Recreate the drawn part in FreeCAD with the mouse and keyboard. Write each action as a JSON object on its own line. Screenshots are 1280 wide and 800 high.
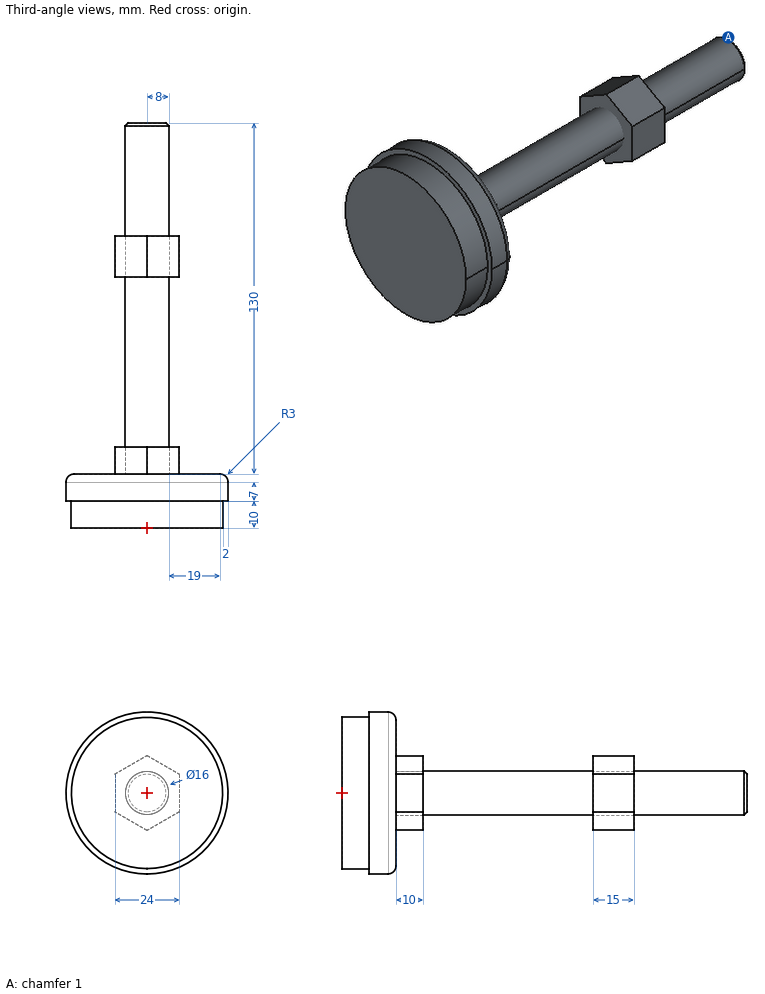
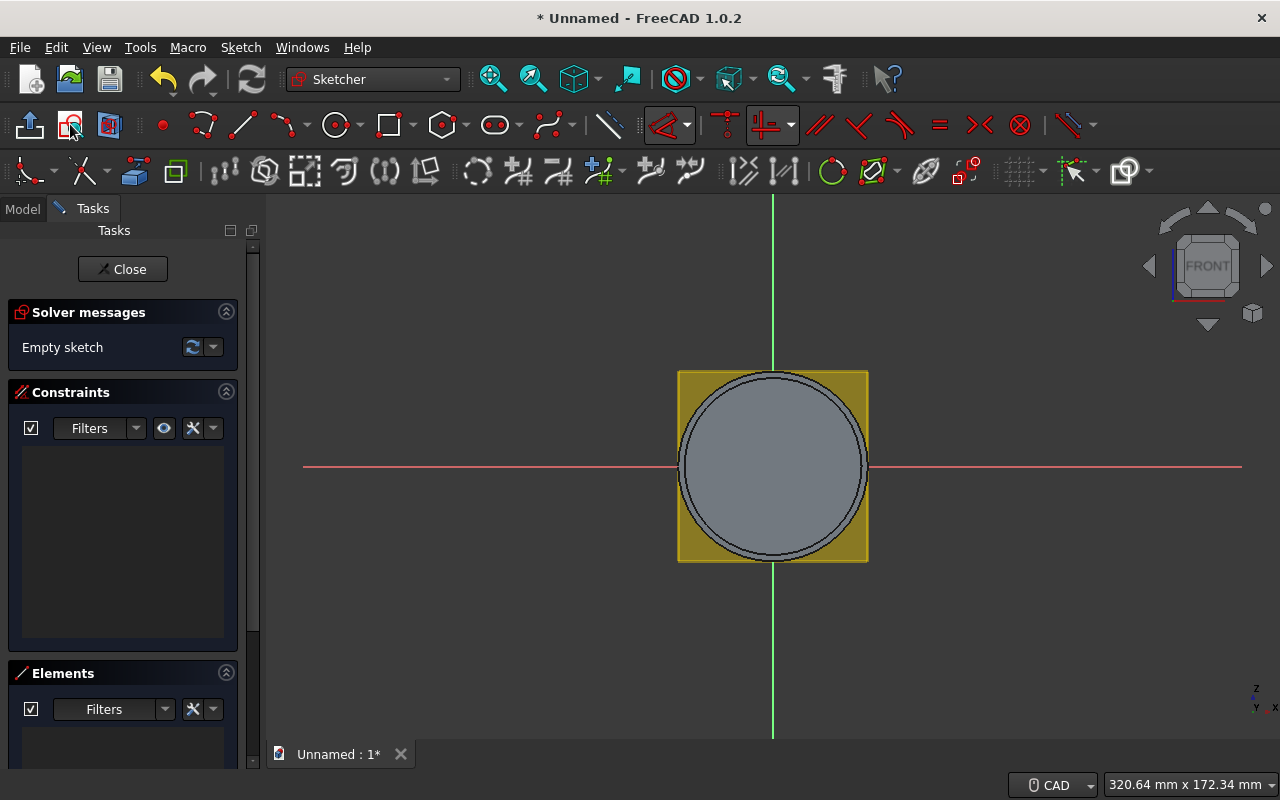
{"action": "scroll", "coordinate": [795, 466], "scroll_direction": "up", "scroll_amount": 7}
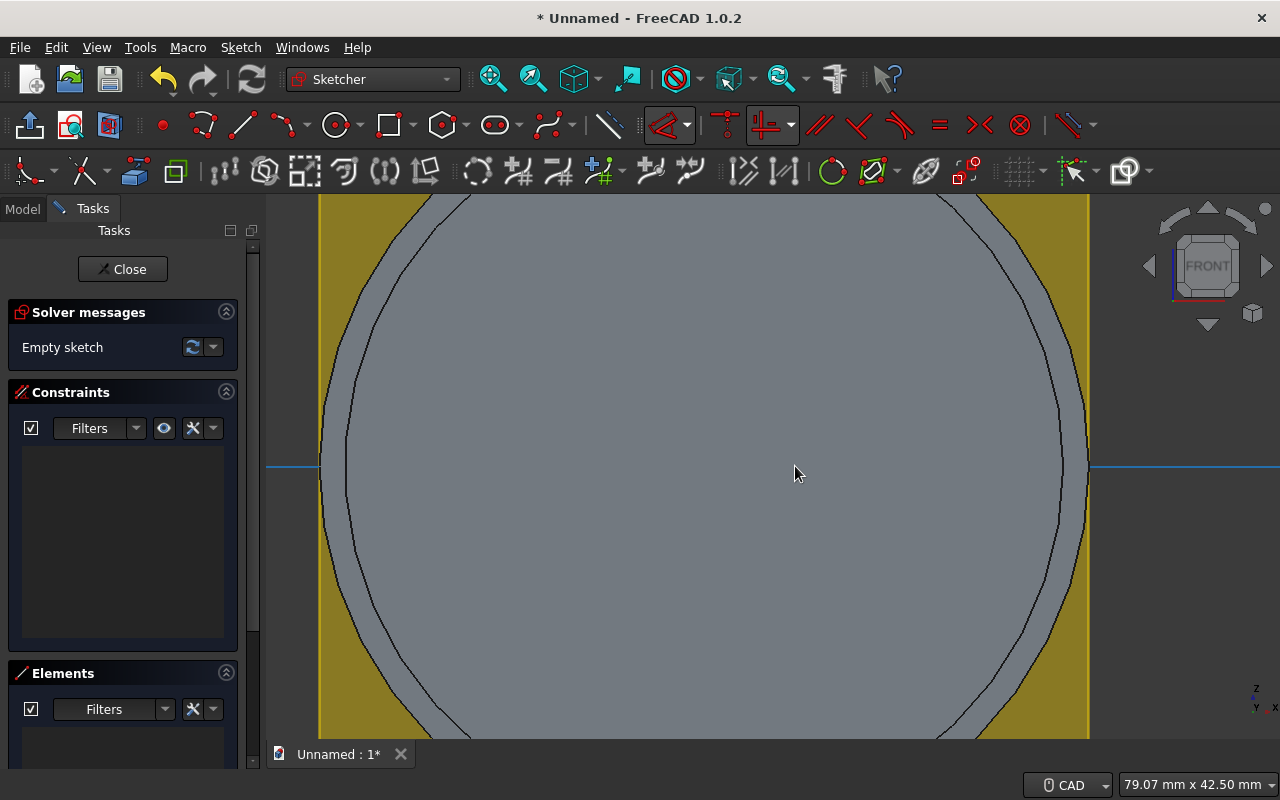
{"action": "left_click", "coordinate": [442, 126]}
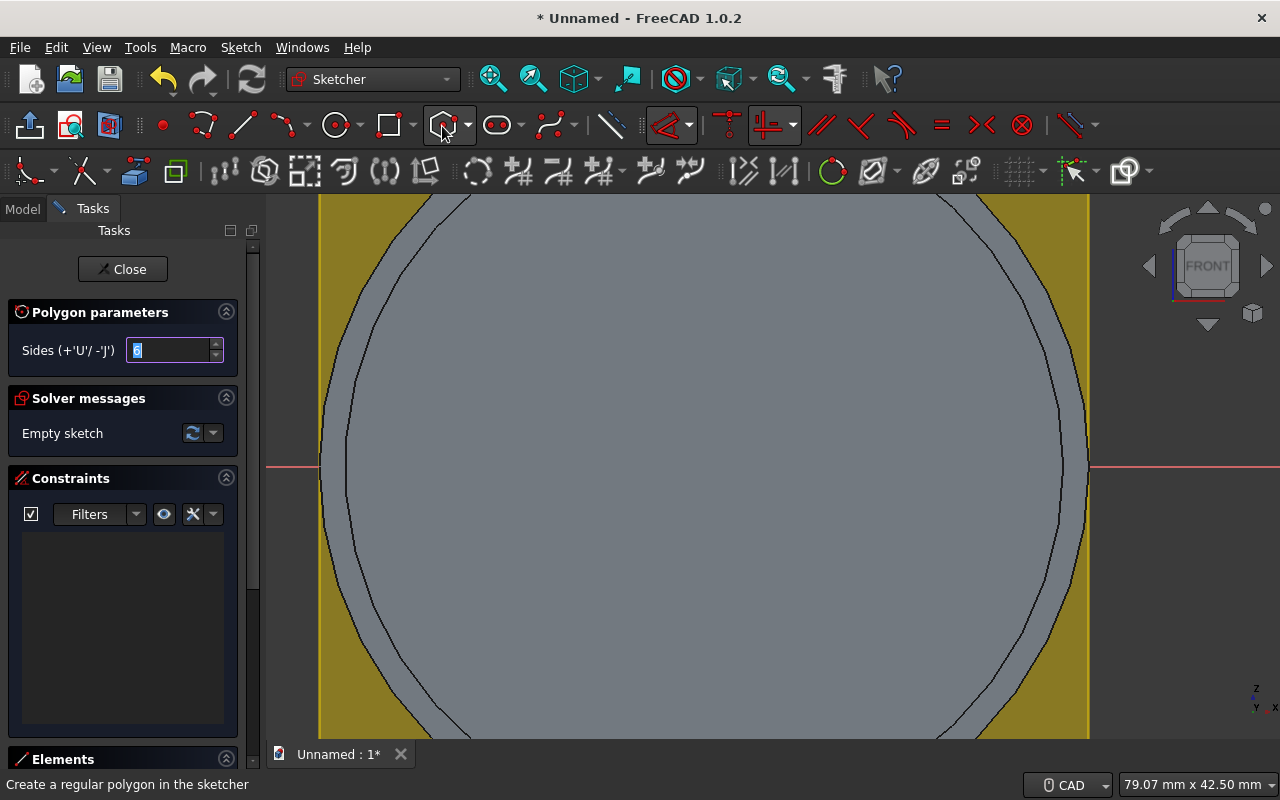
{"action": "left_click", "coordinate": [704, 467]}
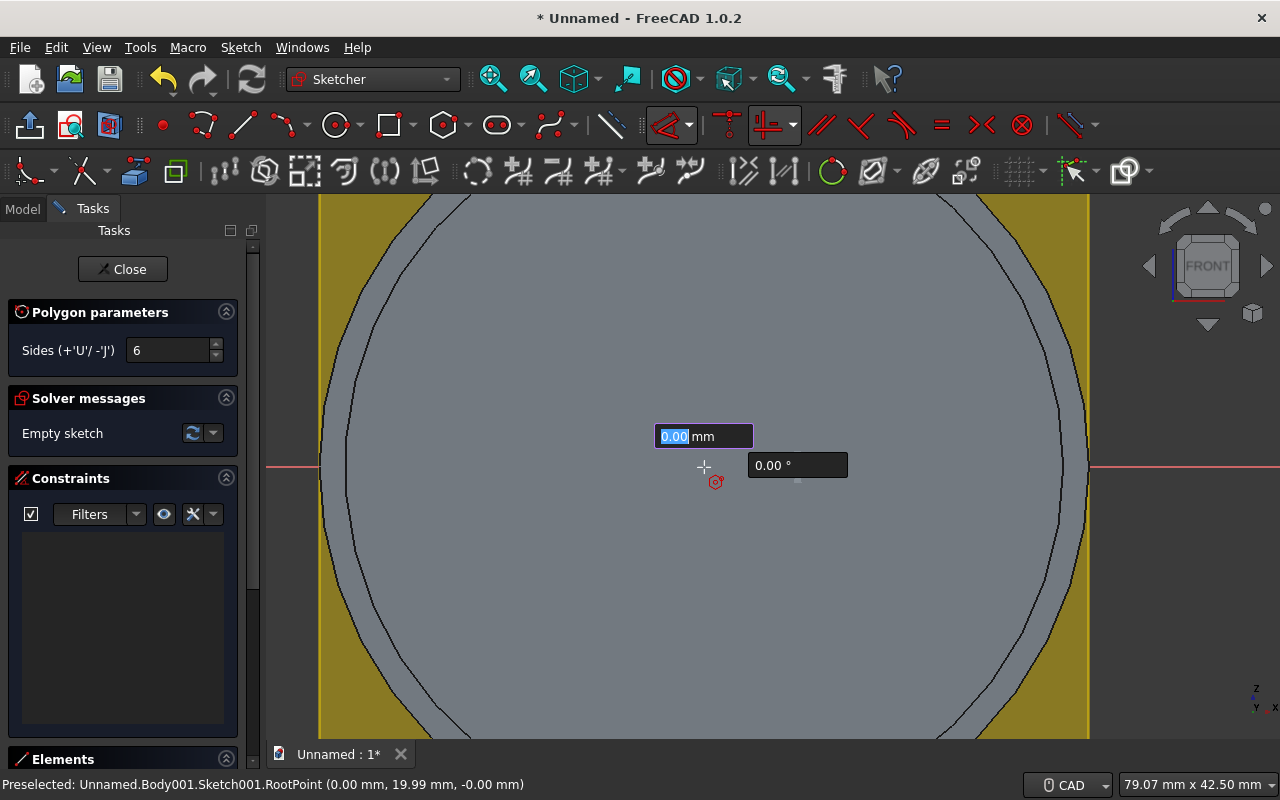
{"action": "left_click", "coordinate": [704, 644]}
{"action": "key", "text": "Escape"}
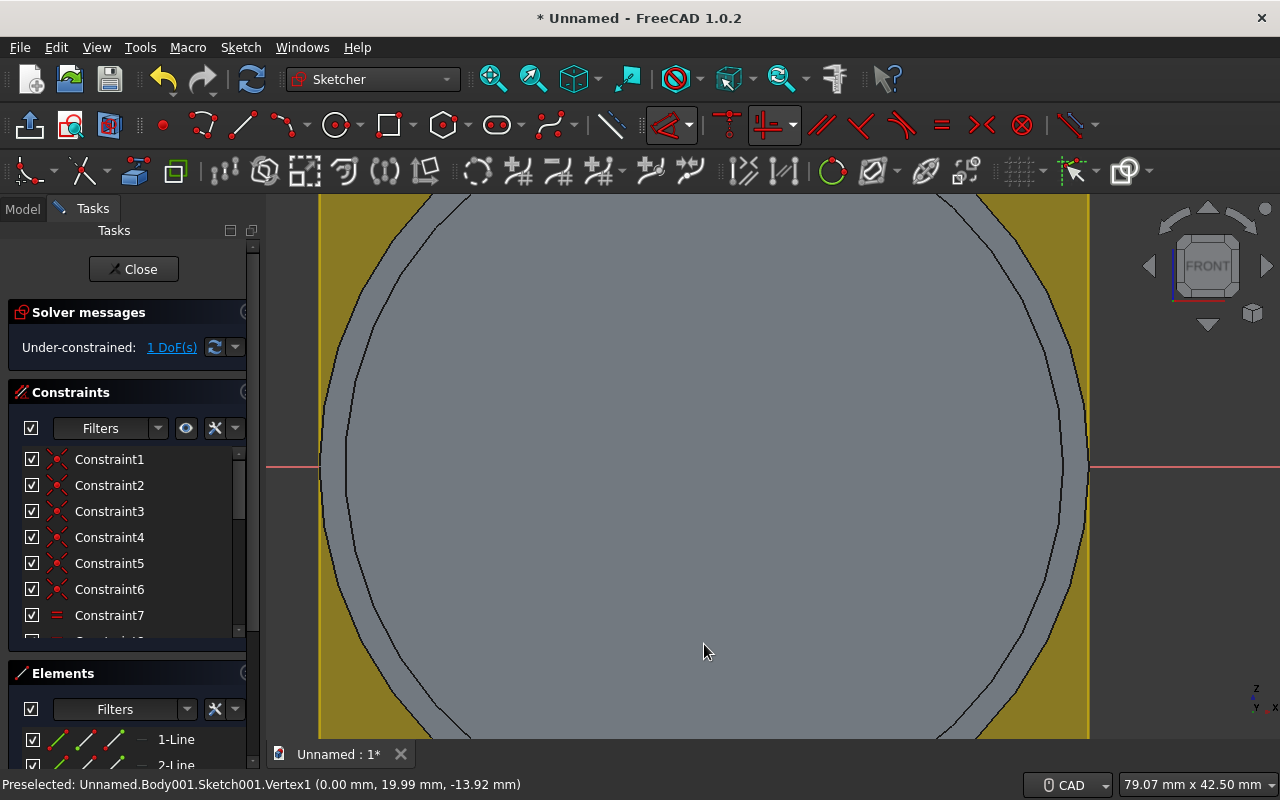
{"action": "left_click", "coordinate": [336, 126]}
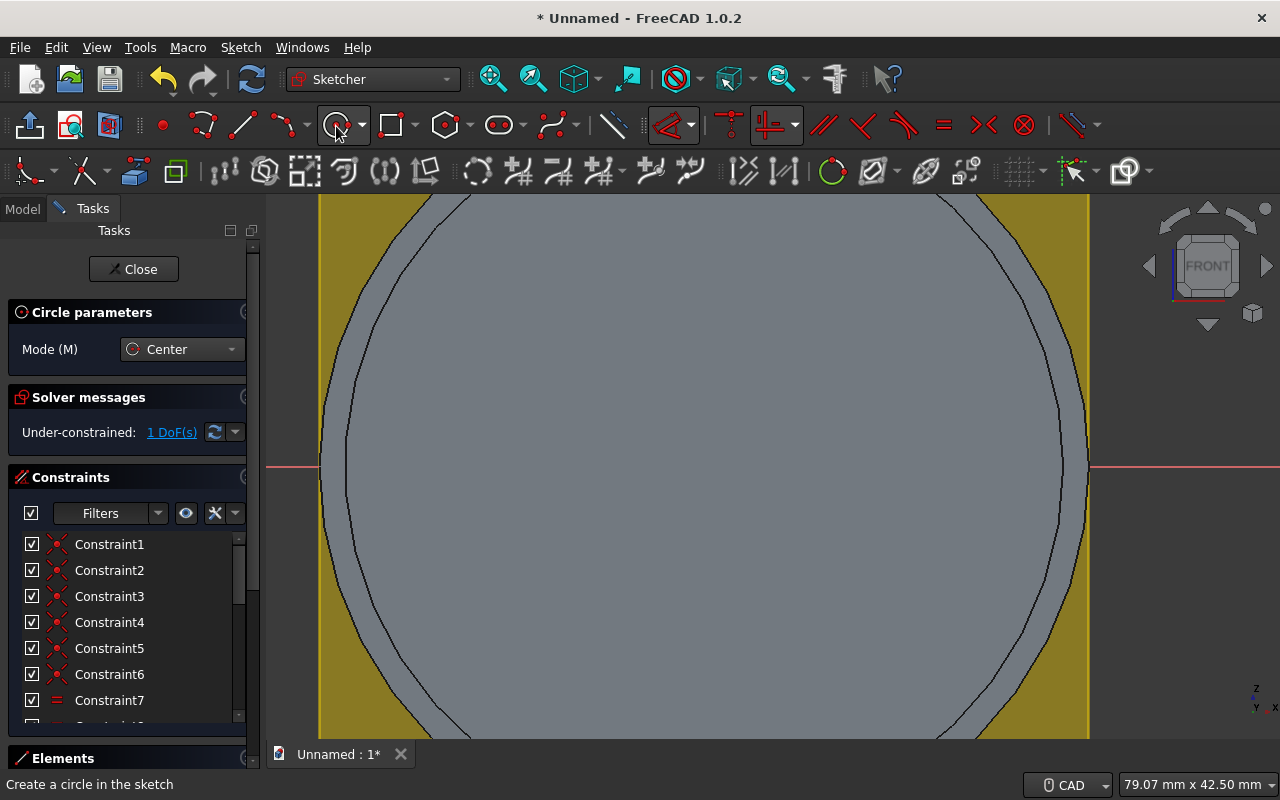
{"action": "left_click", "coordinate": [704, 467]}
{"action": "left_click", "coordinate": [777, 394]}
{"action": "key", "text": "Escape"}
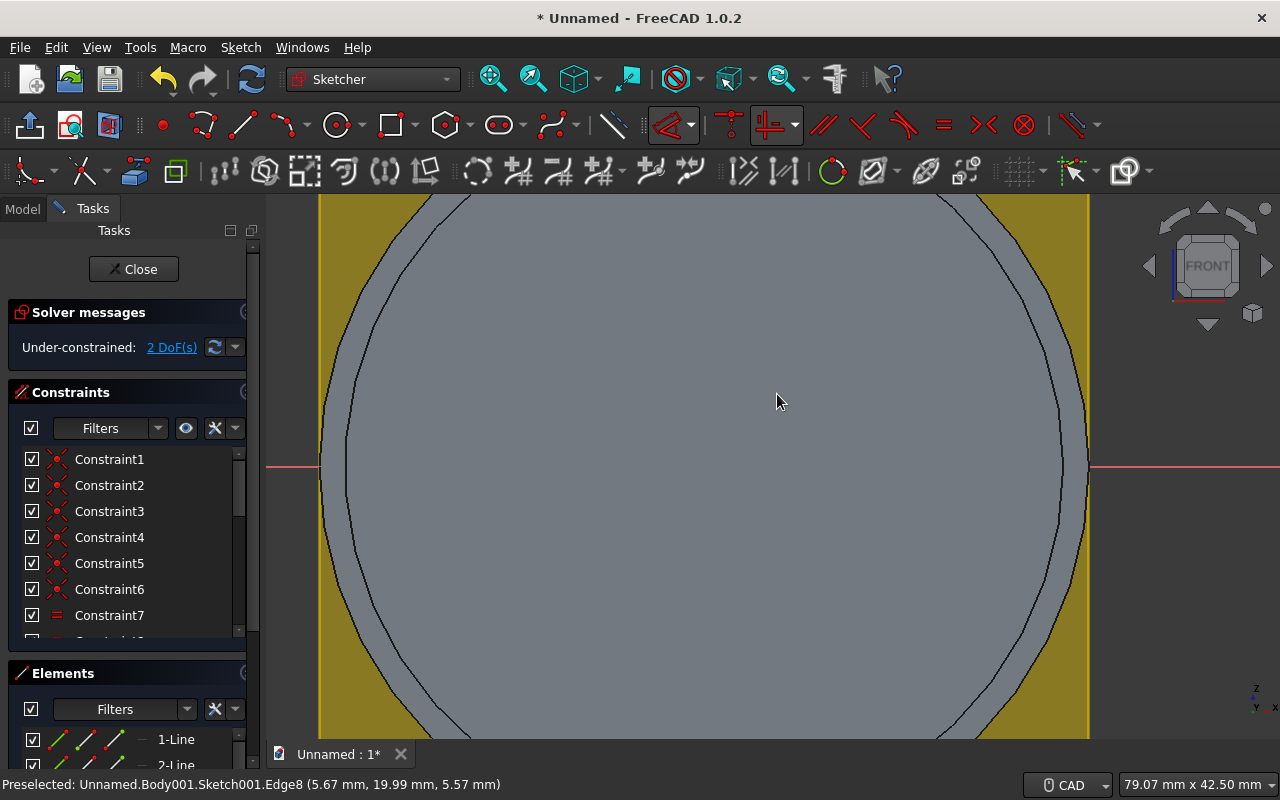
{"action": "left_click", "coordinate": [776, 394]}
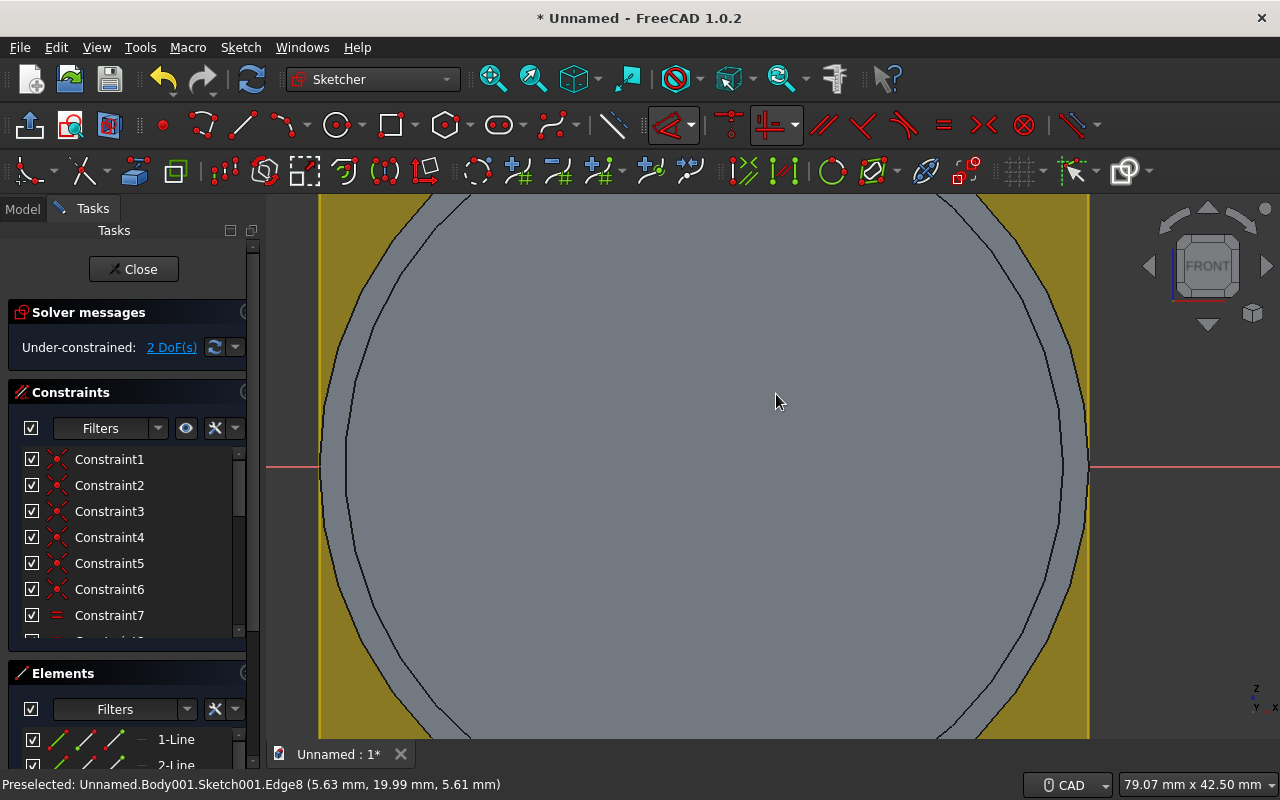
{"action": "left_click", "coordinate": [694, 126]}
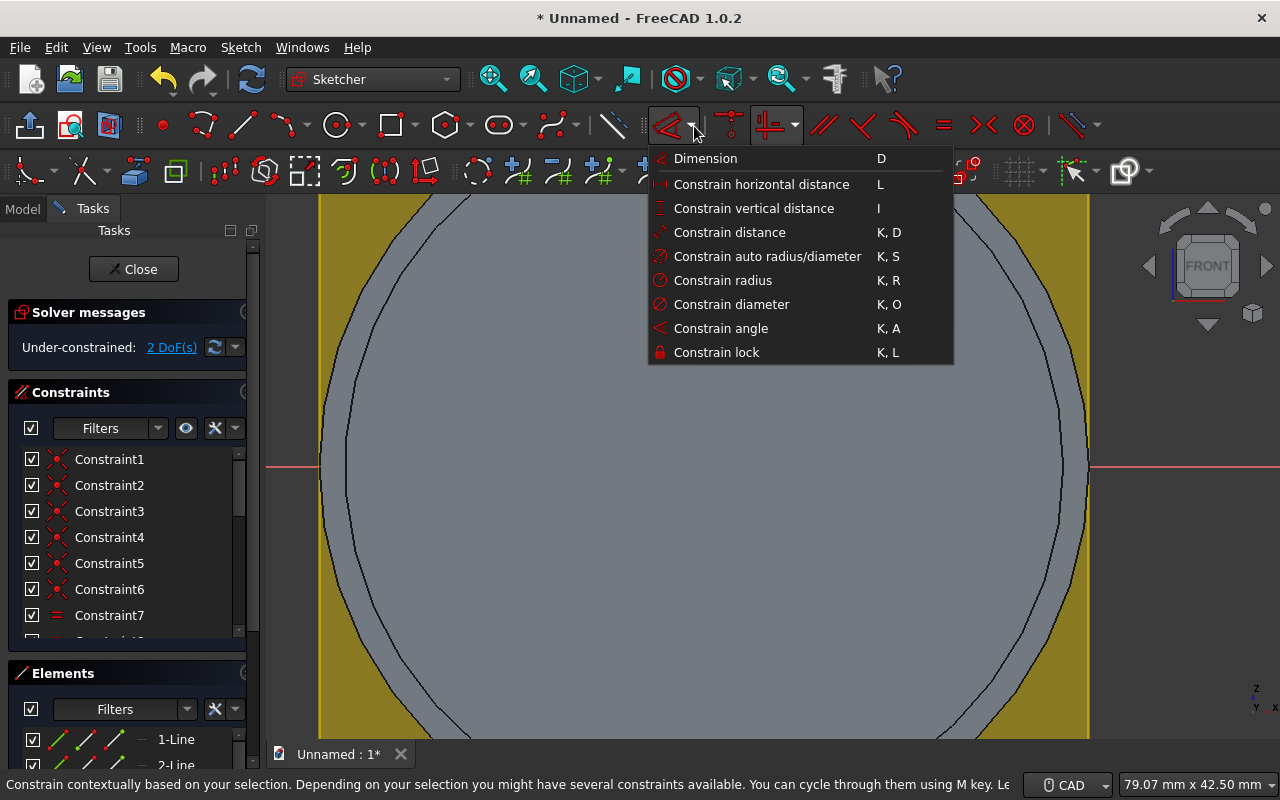
{"action": "left_click", "coordinate": [801, 304]}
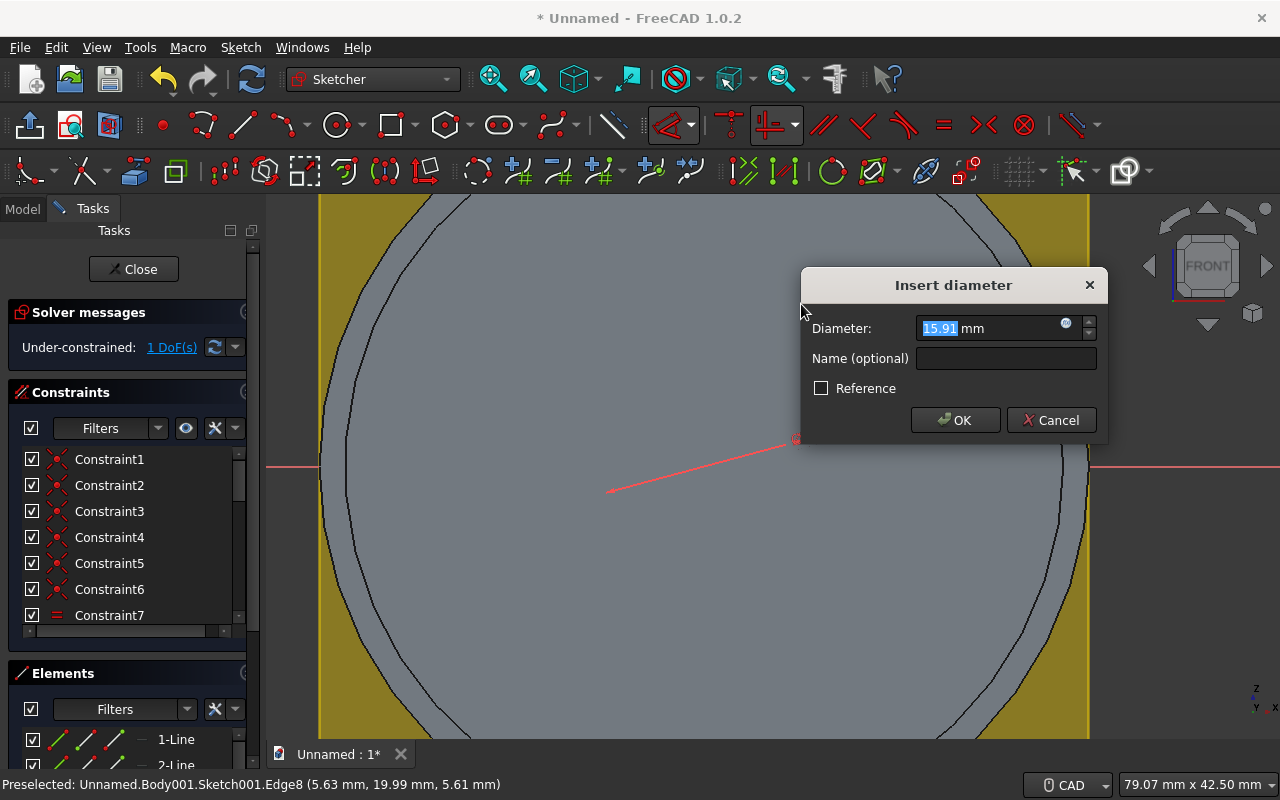
{"action": "type", "text": "16"}
{"action": "key", "text": "Return"}